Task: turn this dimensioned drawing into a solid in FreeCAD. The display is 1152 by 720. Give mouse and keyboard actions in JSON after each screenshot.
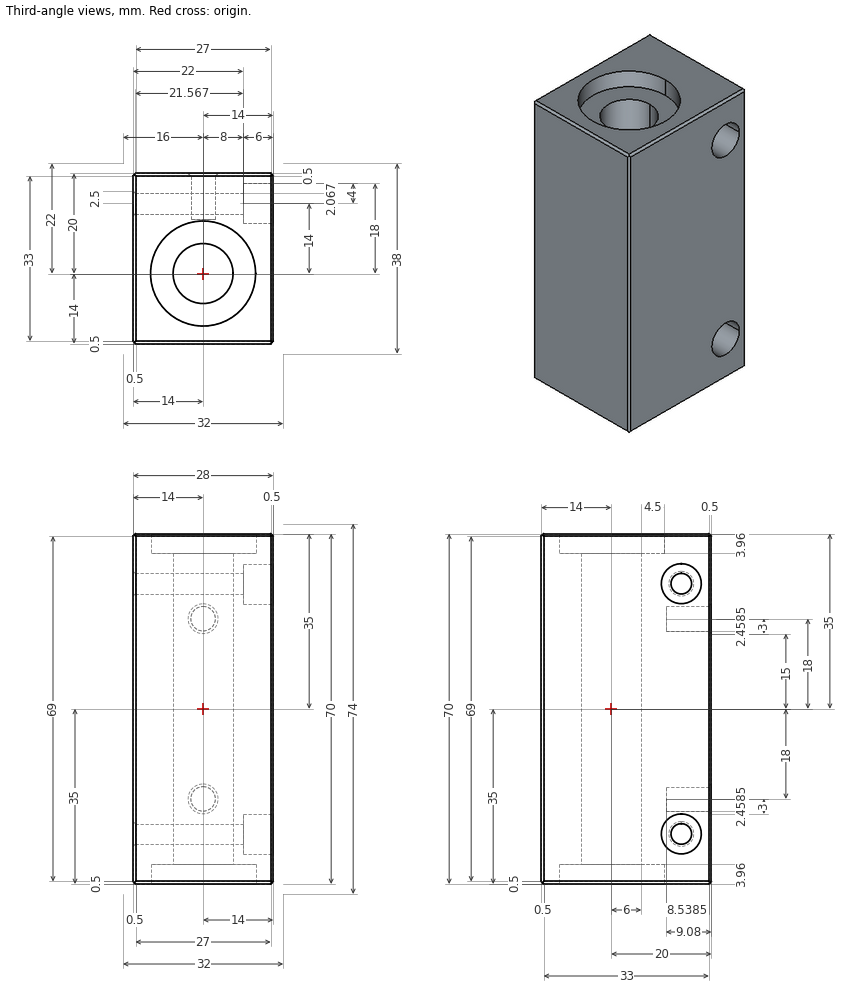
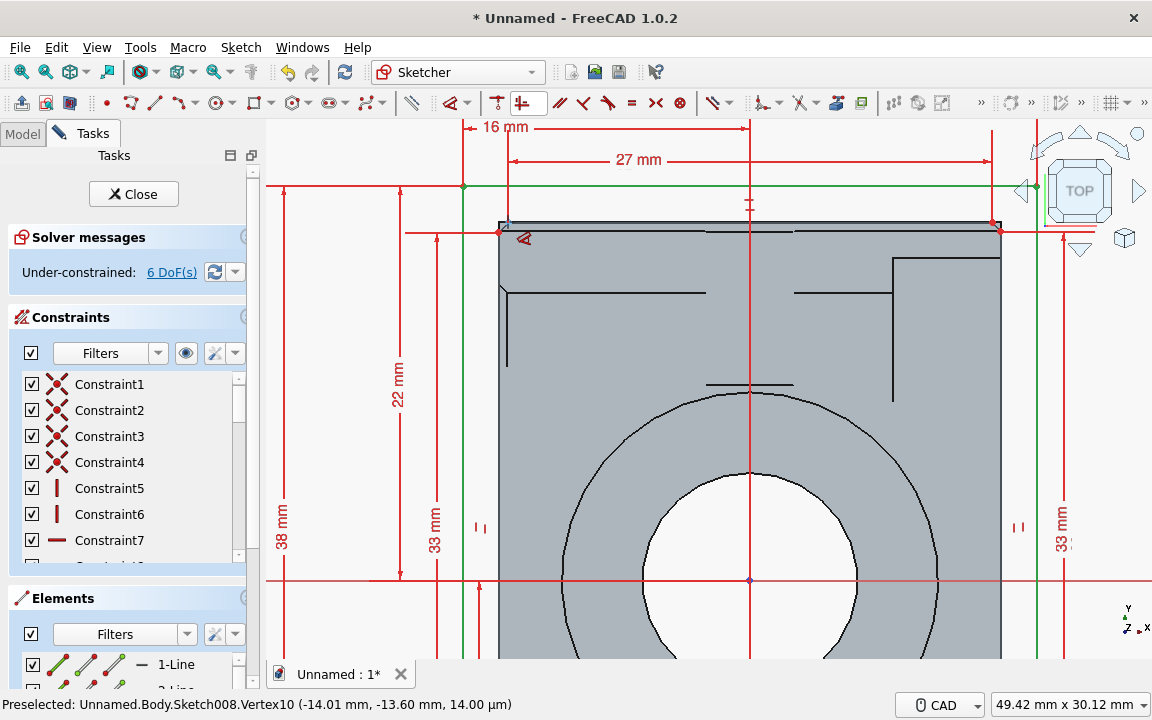
{"action": "left_click", "coordinate": [508, 223]}
{"action": "left_click", "coordinate": [784, 402]}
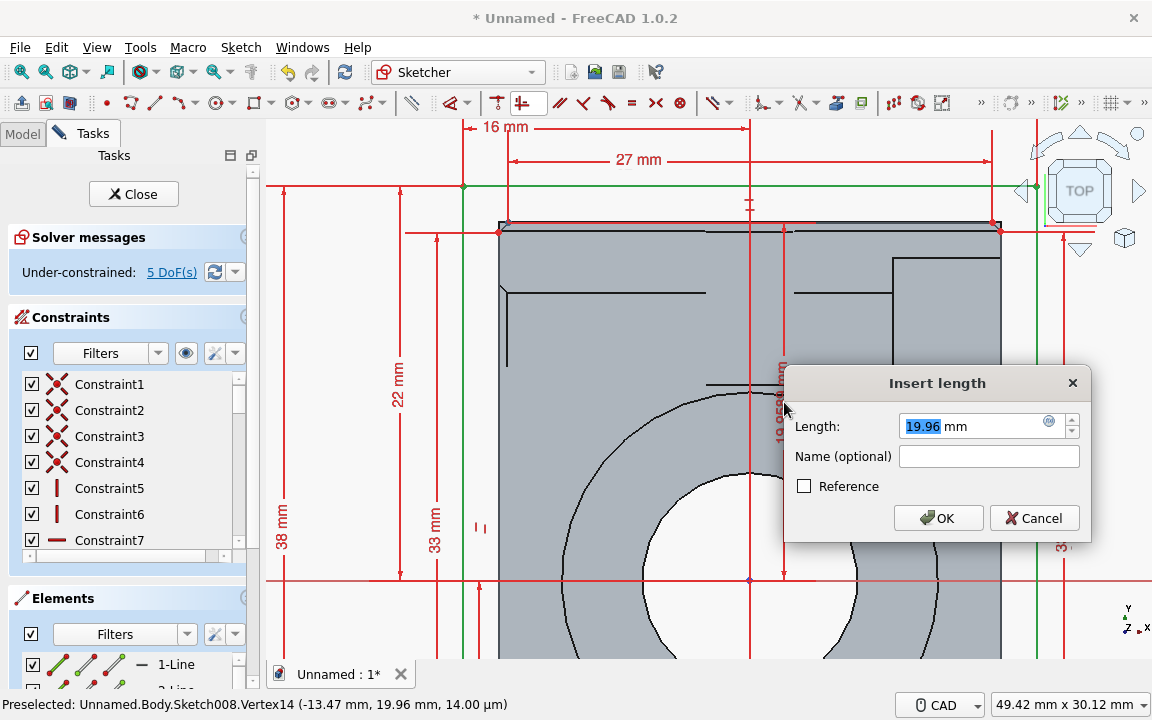
{"action": "type", "text": "20"}
{"action": "key", "text": "Return"}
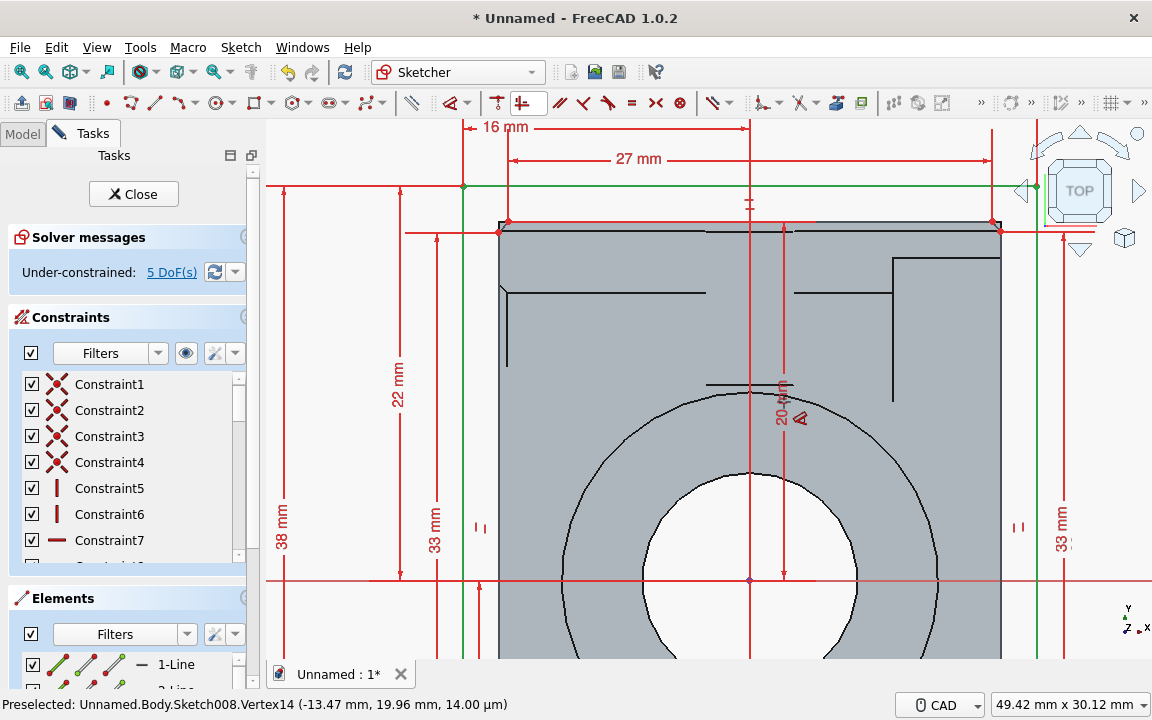
{"action": "scroll", "coordinate": [507, 221], "scroll_direction": "down", "scroll_amount": 3}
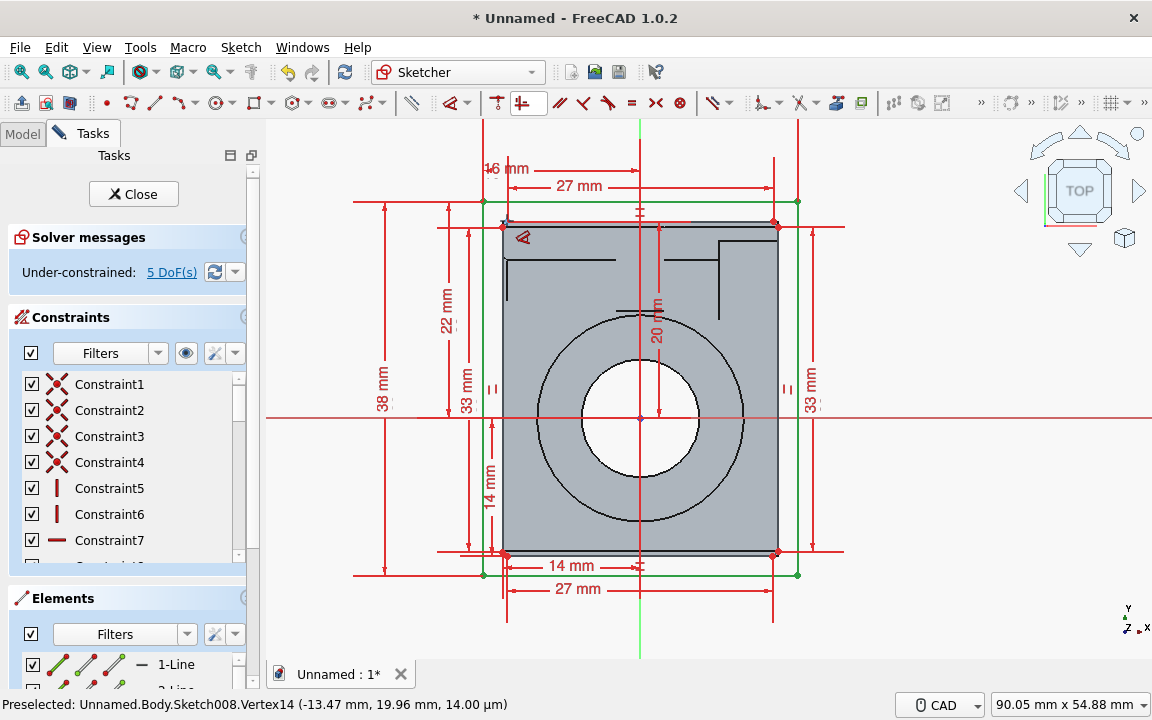
{"action": "scroll", "coordinate": [778, 227], "scroll_direction": "up", "scroll_amount": 3}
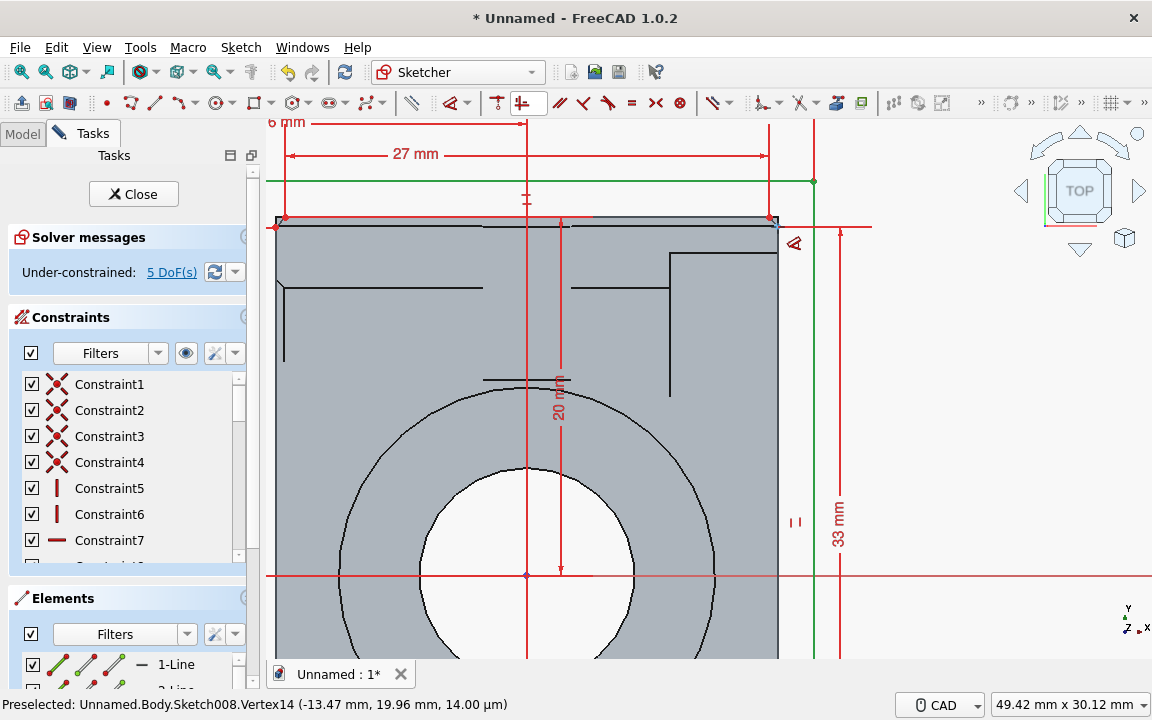
{"action": "left_click", "coordinate": [778, 227]}
{"action": "left_click", "coordinate": [652, 610]}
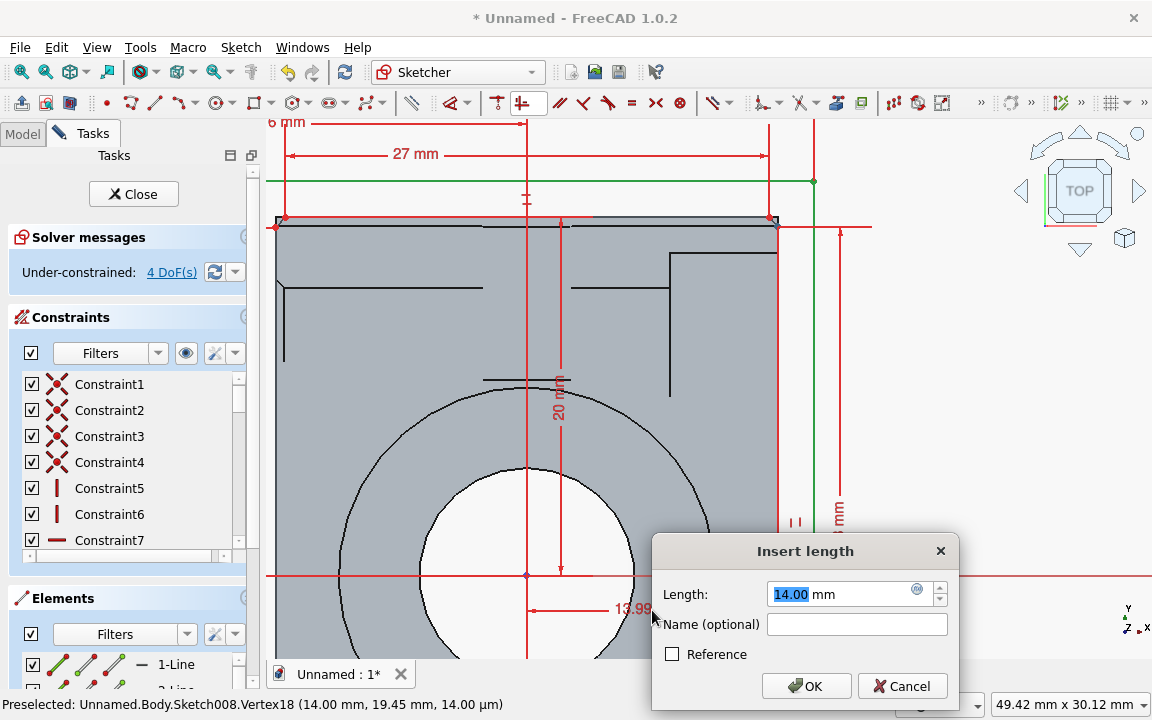
{"action": "type", "text": "14"}
{"action": "key", "text": "Return"}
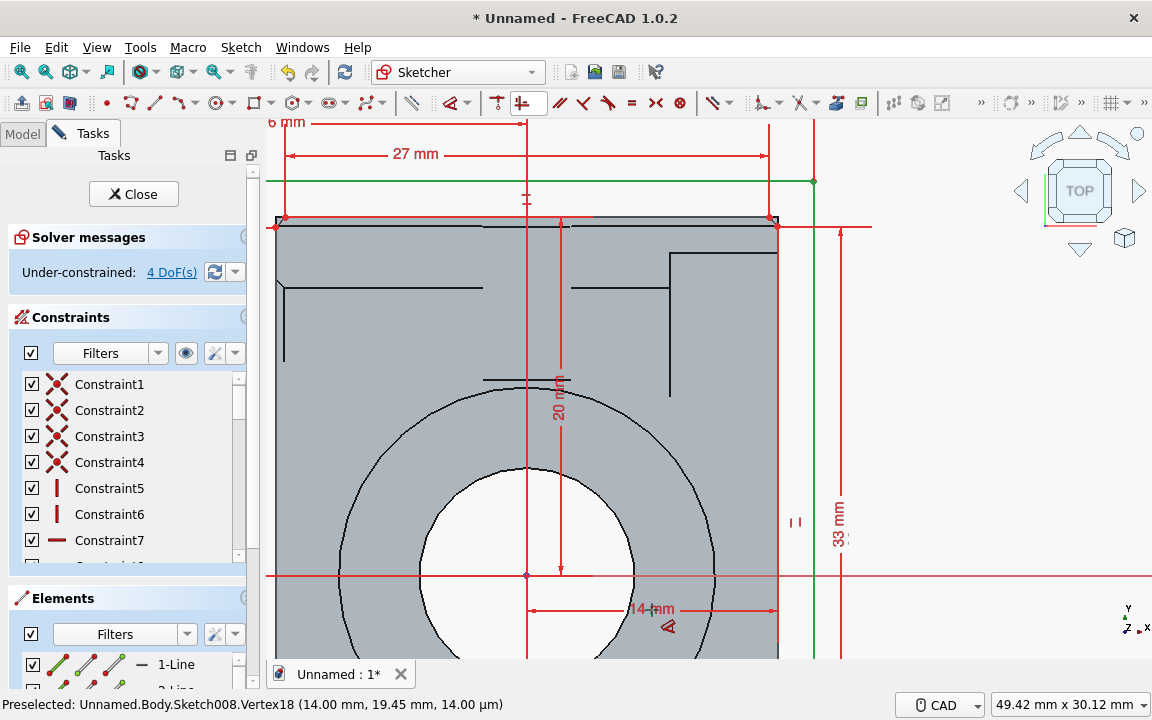
{"action": "scroll", "coordinate": [779, 227], "scroll_direction": "down", "scroll_amount": 3}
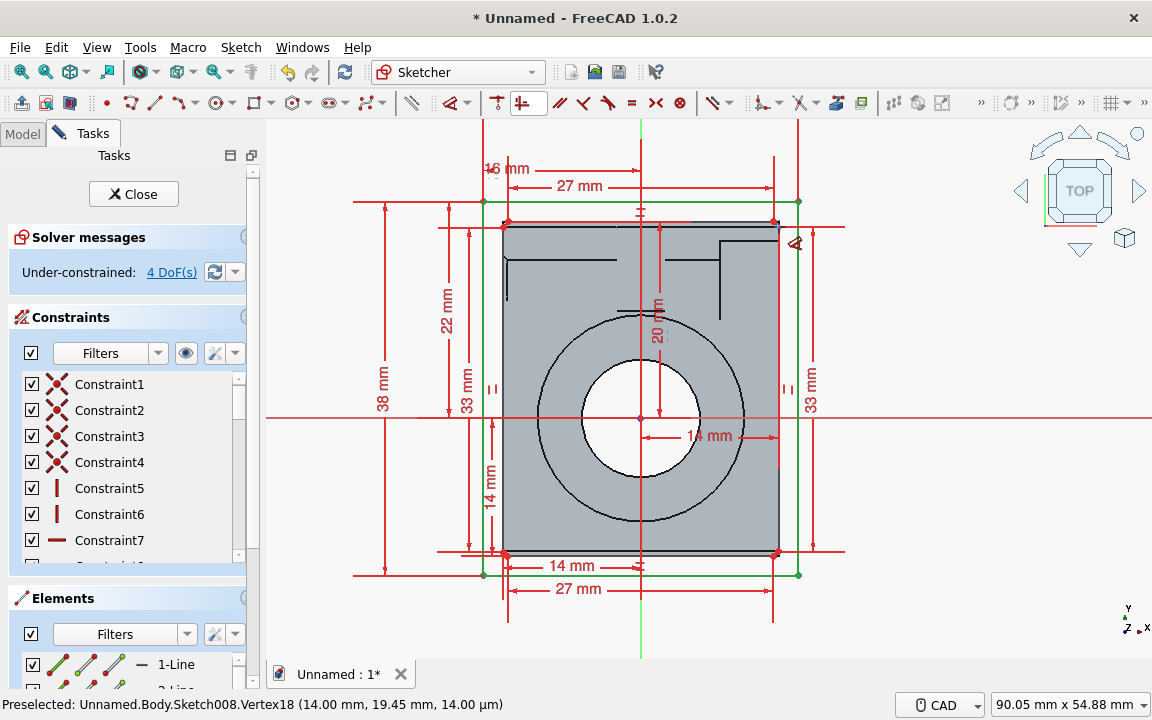
{"action": "scroll", "coordinate": [505, 554], "scroll_direction": "up", "scroll_amount": 11}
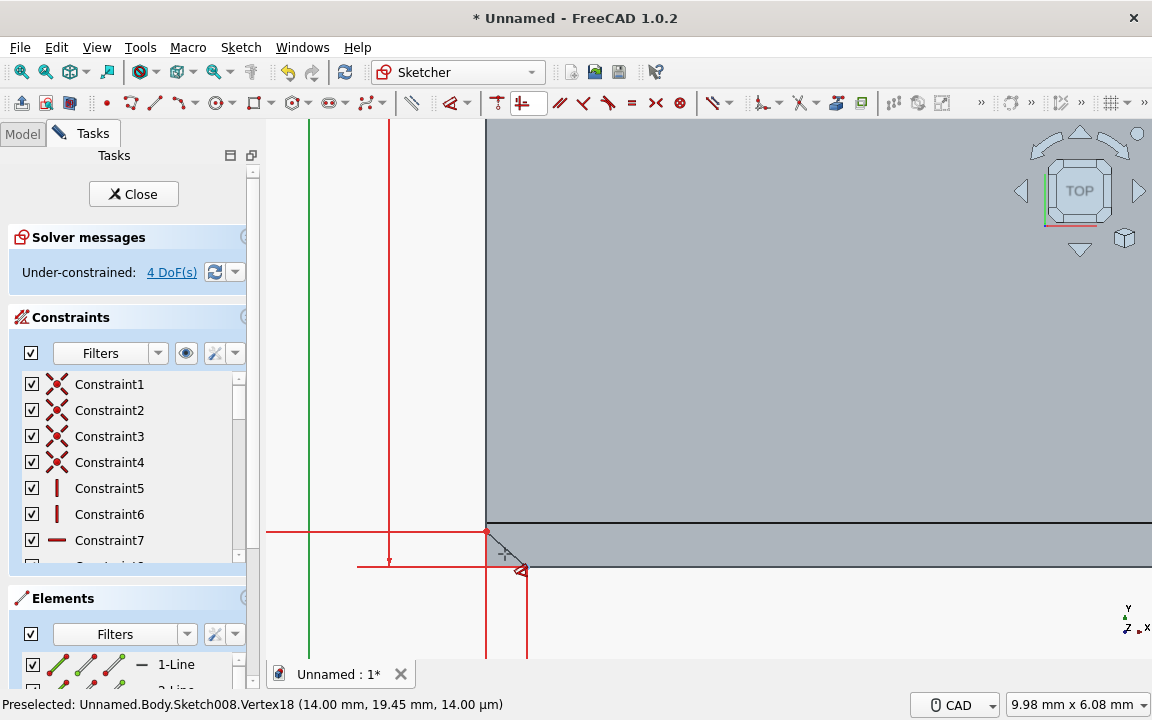
{"action": "left_click", "coordinate": [506, 549]}
{"action": "left_click", "coordinate": [506, 601]}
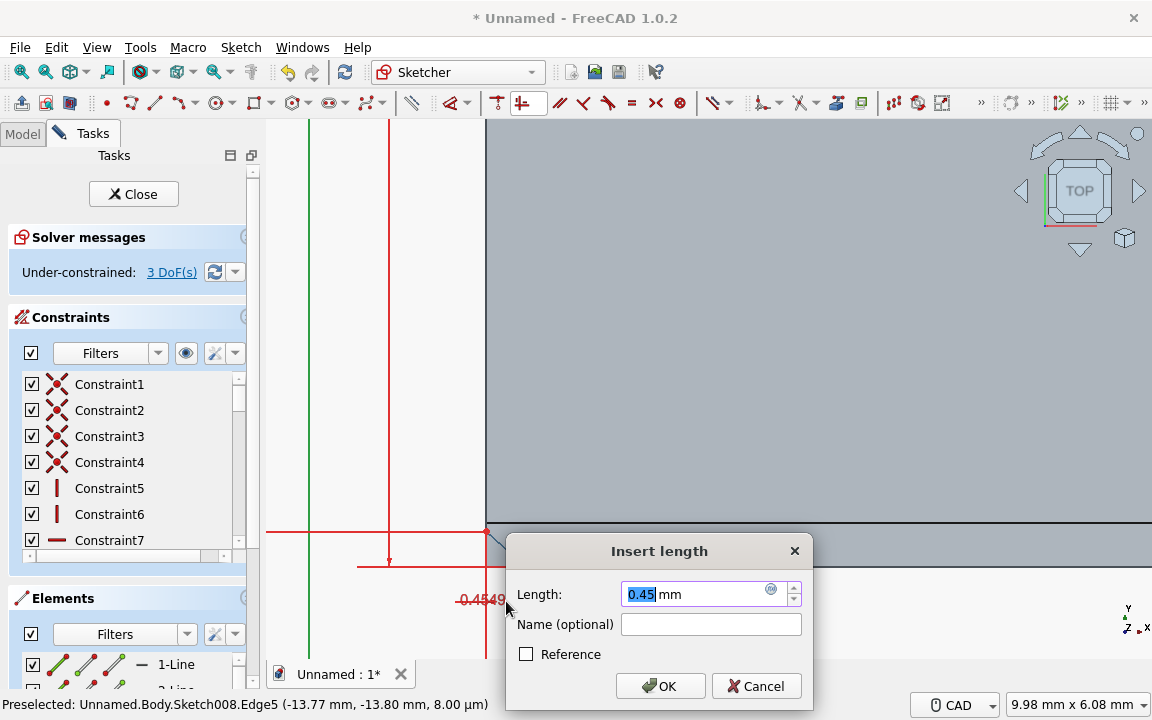
{"action": "type", "text": "0.5"}
{"action": "key", "text": "Return"}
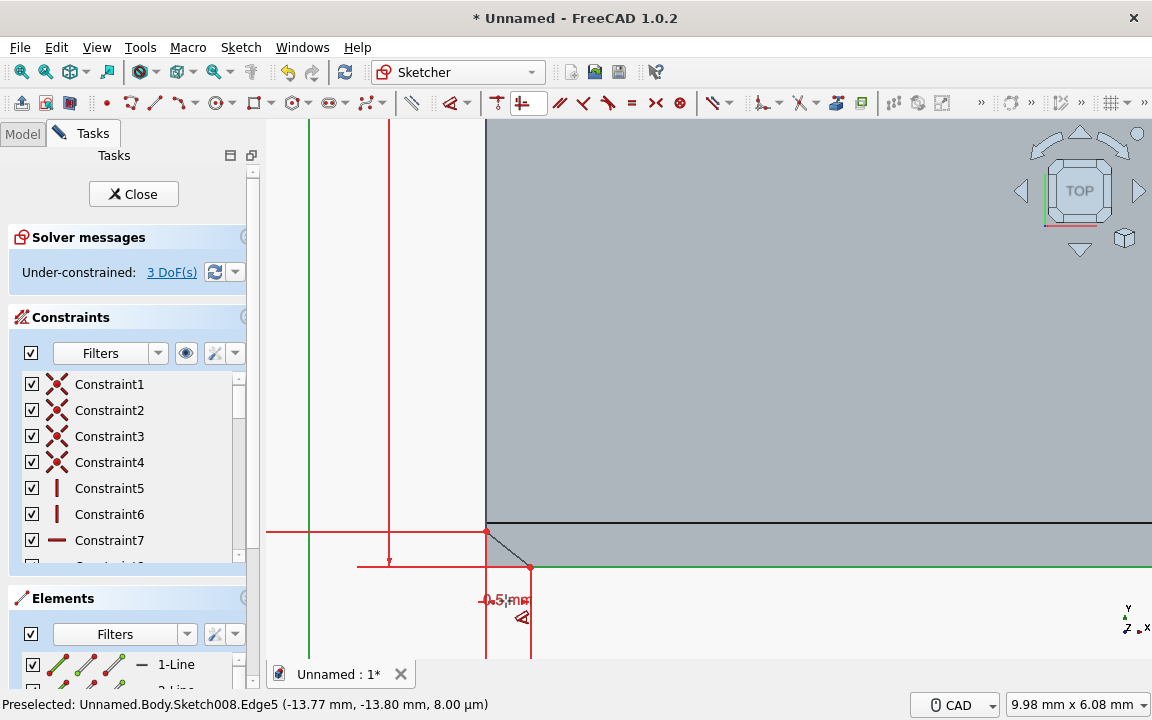
{"action": "left_click", "coordinate": [517, 557]}
{"action": "left_click", "coordinate": [452, 549]}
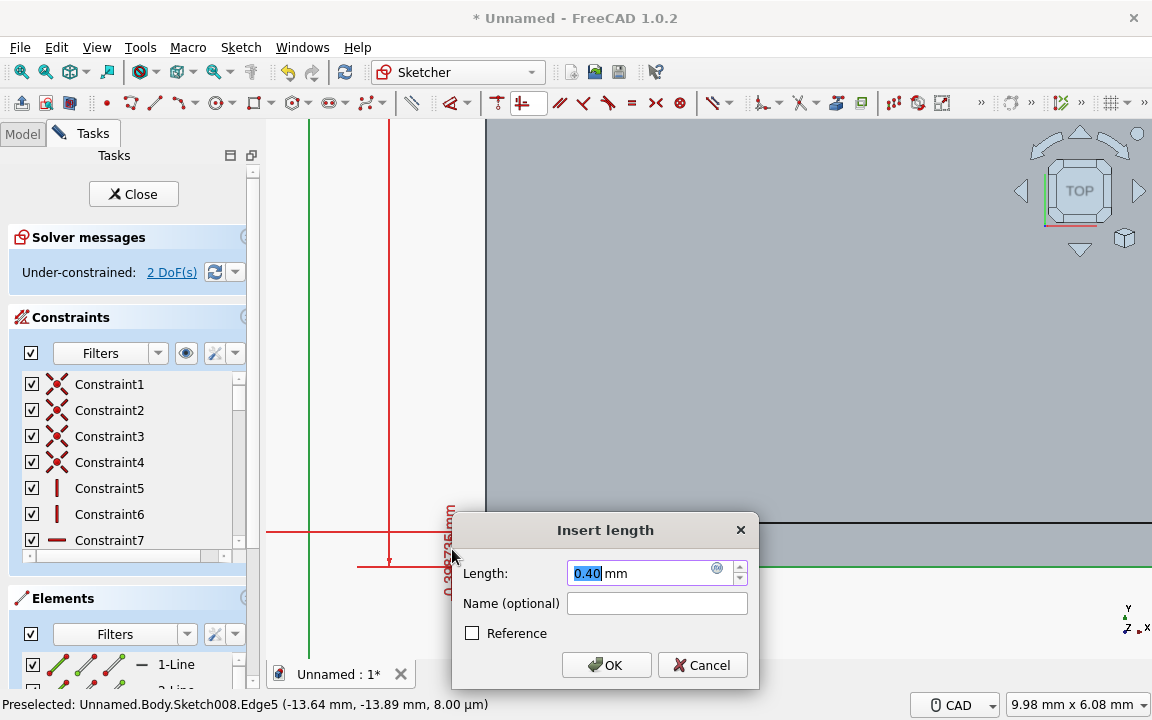
{"action": "type", "text": "0.5"}
{"action": "key", "text": "Return"}